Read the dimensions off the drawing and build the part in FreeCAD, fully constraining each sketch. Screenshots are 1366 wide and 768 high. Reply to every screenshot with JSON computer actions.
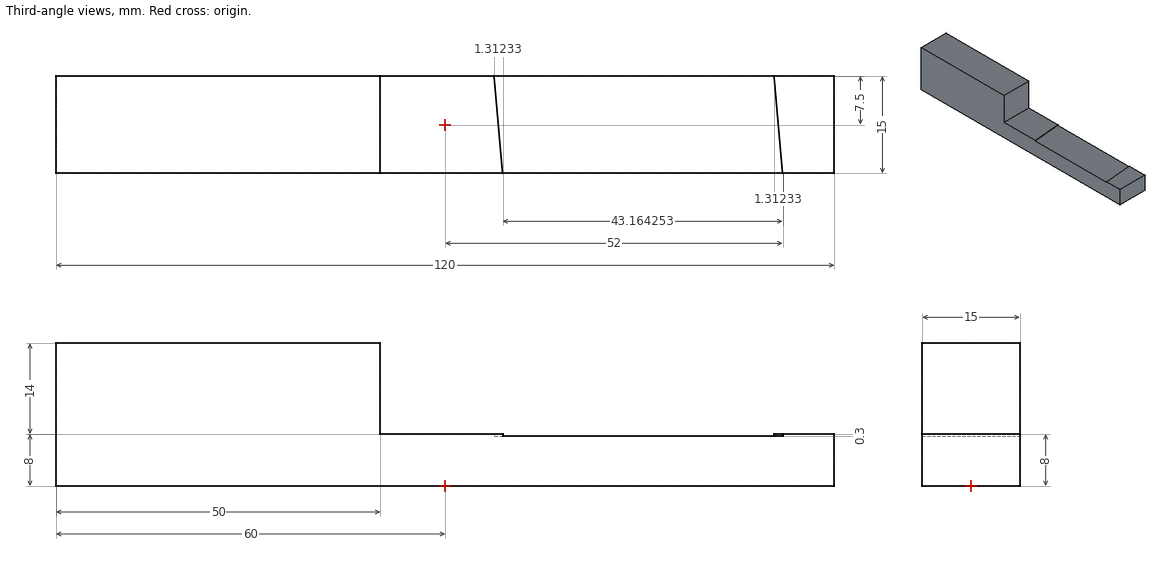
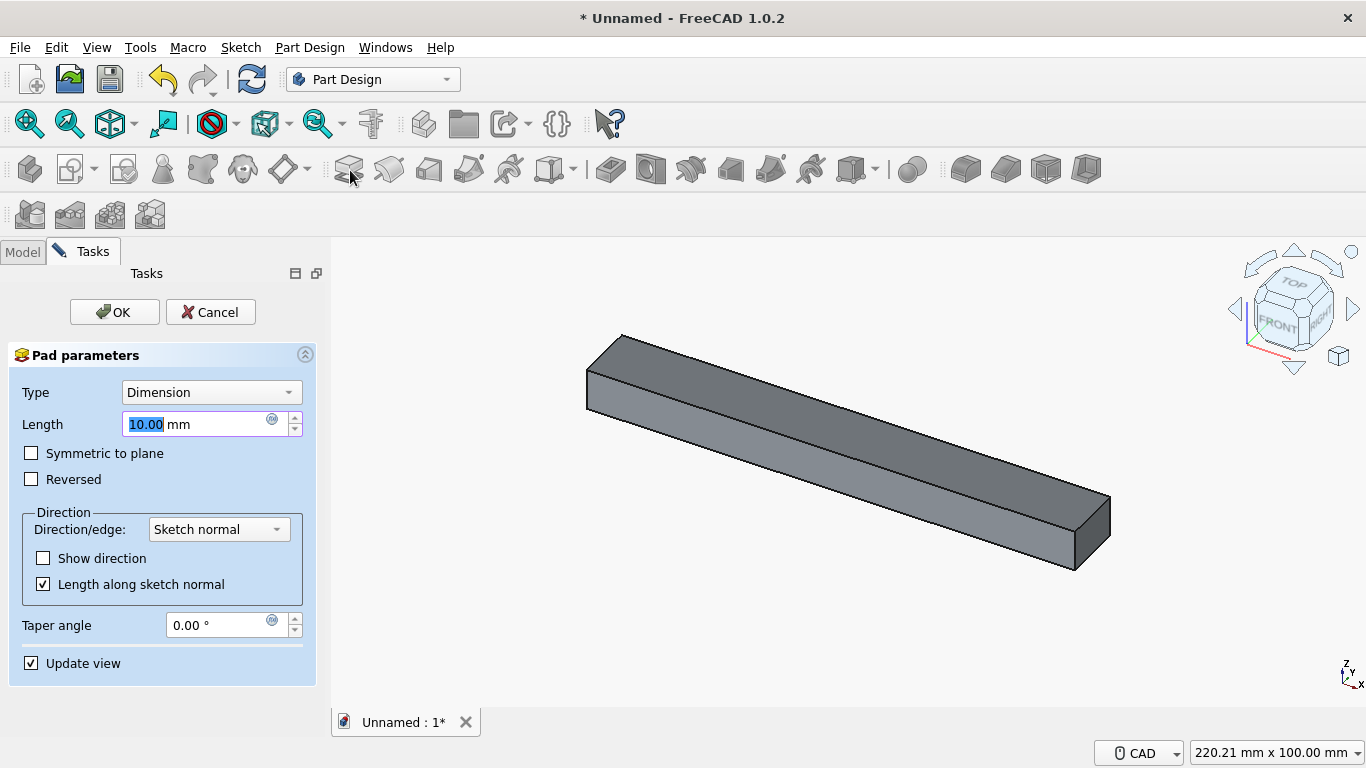
{"action": "type", "text": "8"}
{"action": "key", "text": "Tab"}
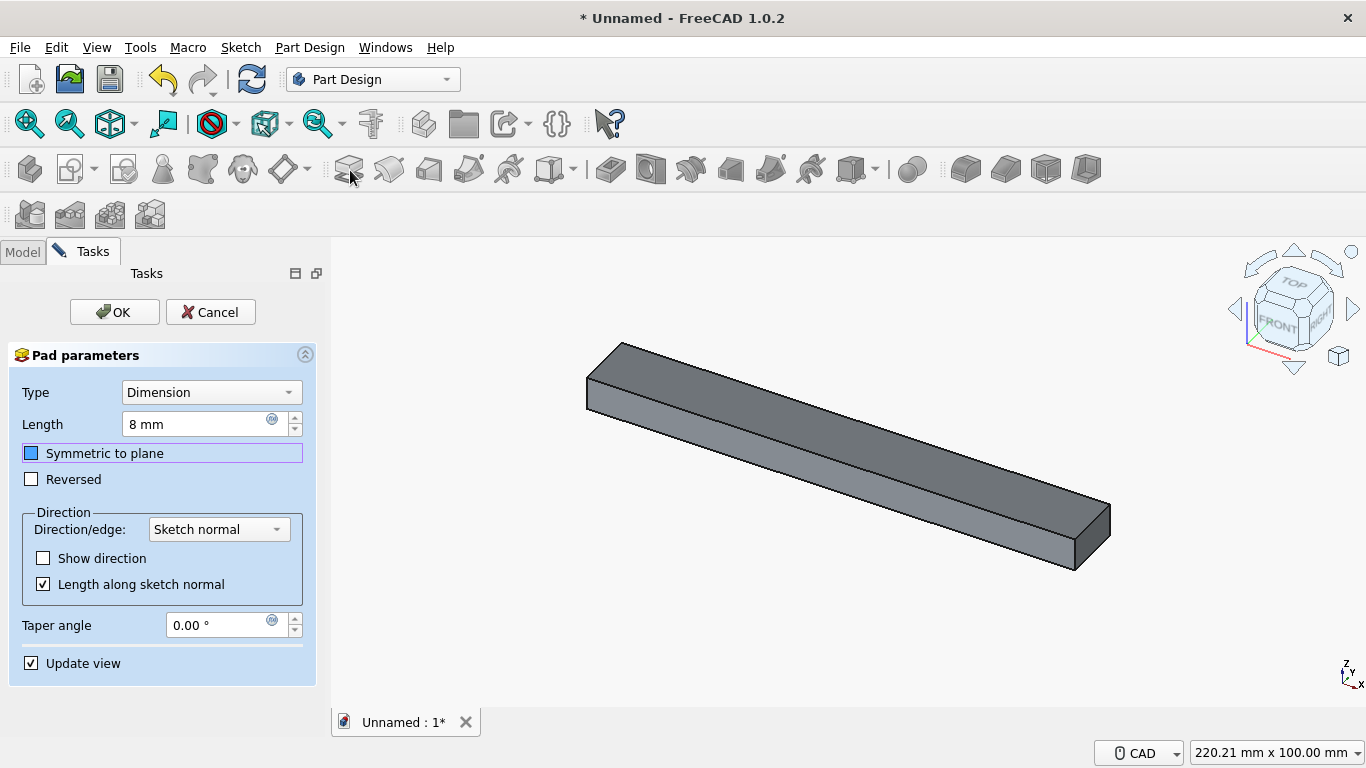
{"action": "left_click", "coordinate": [115, 312]}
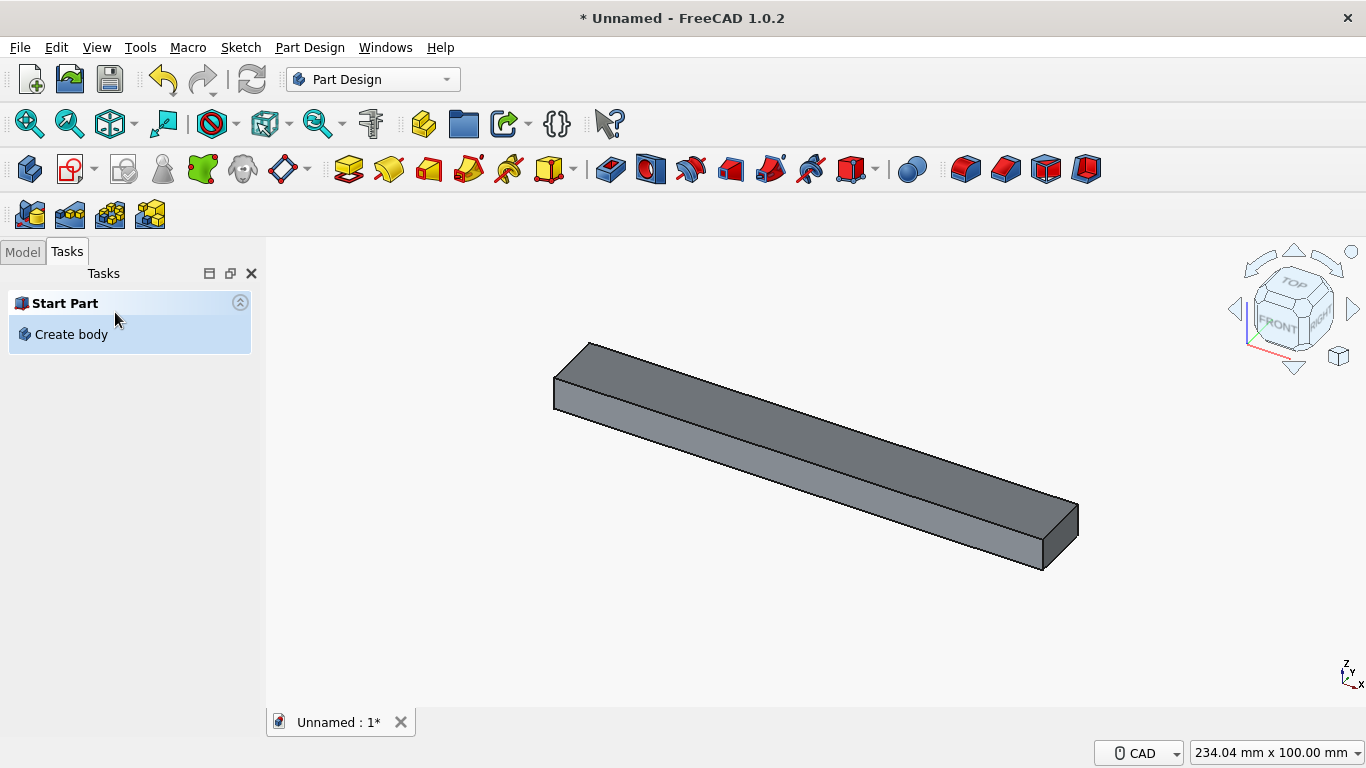
{"action": "left_click", "coordinate": [1025, 510]}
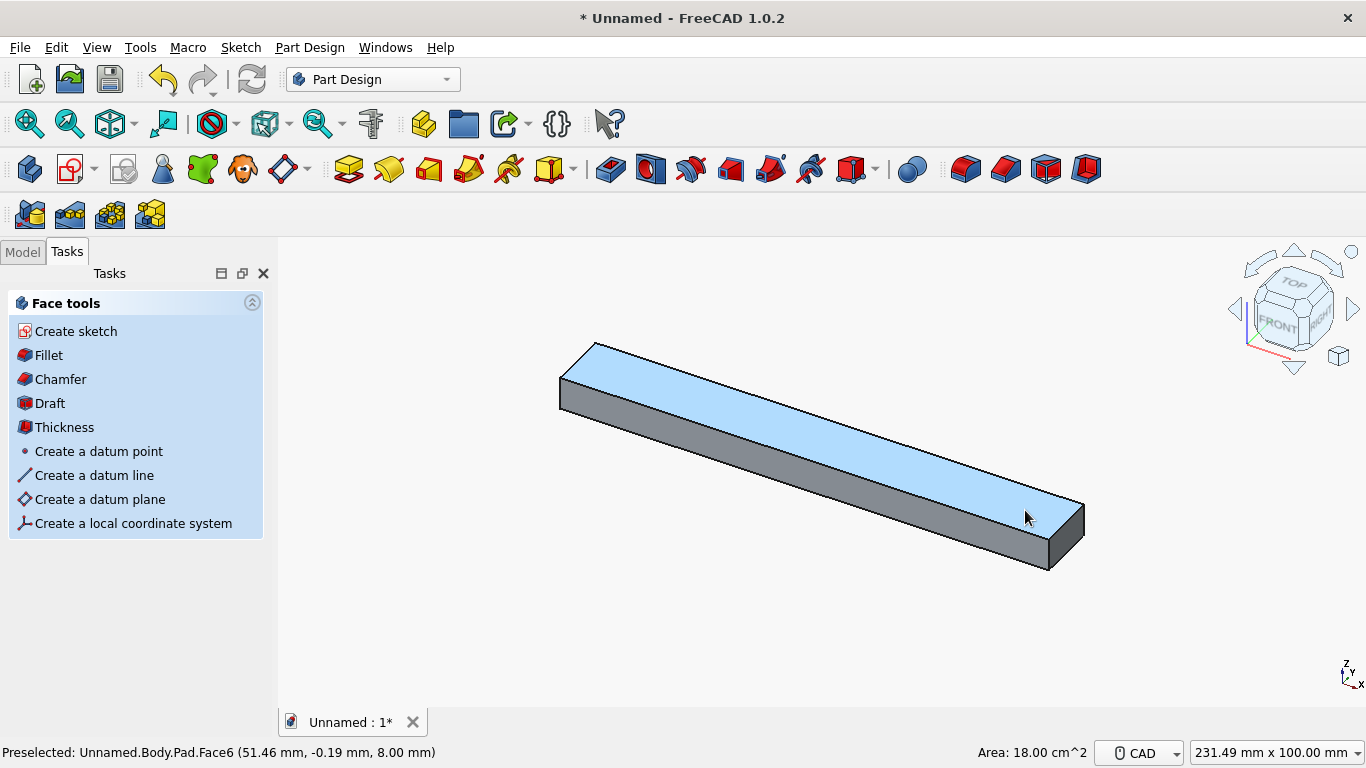
{"action": "left_click", "coordinate": [70, 170]}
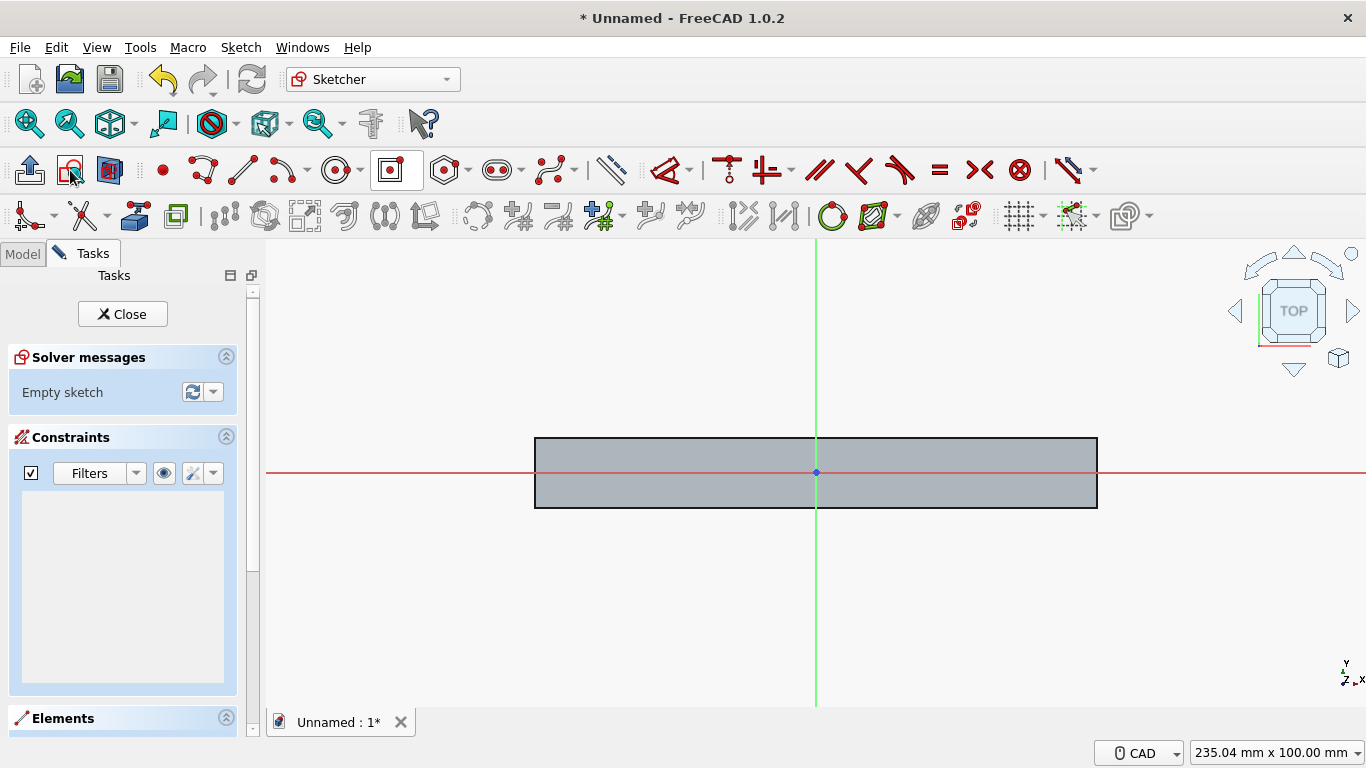
{"action": "scroll", "coordinate": [1048, 473], "scroll_direction": "up", "scroll_amount": 5}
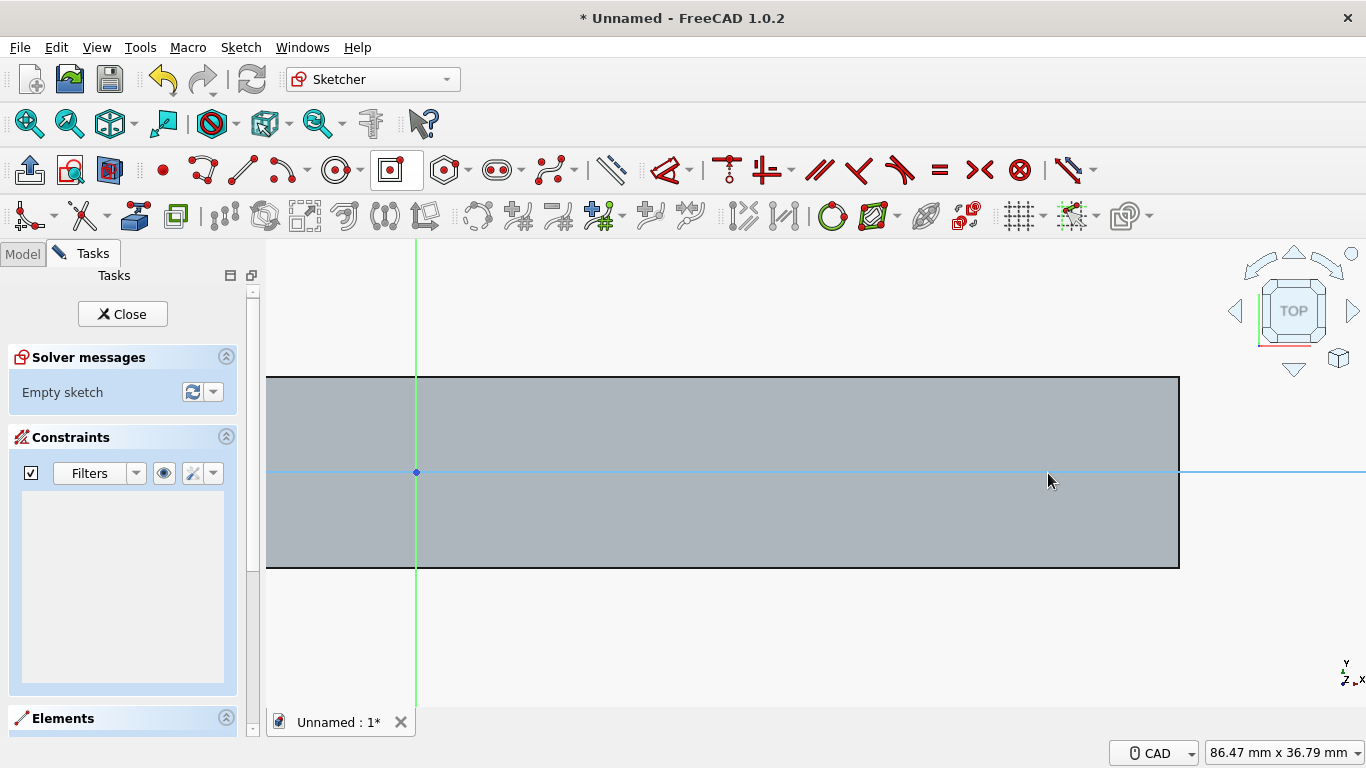
{"action": "left_click", "coordinate": [204, 170]}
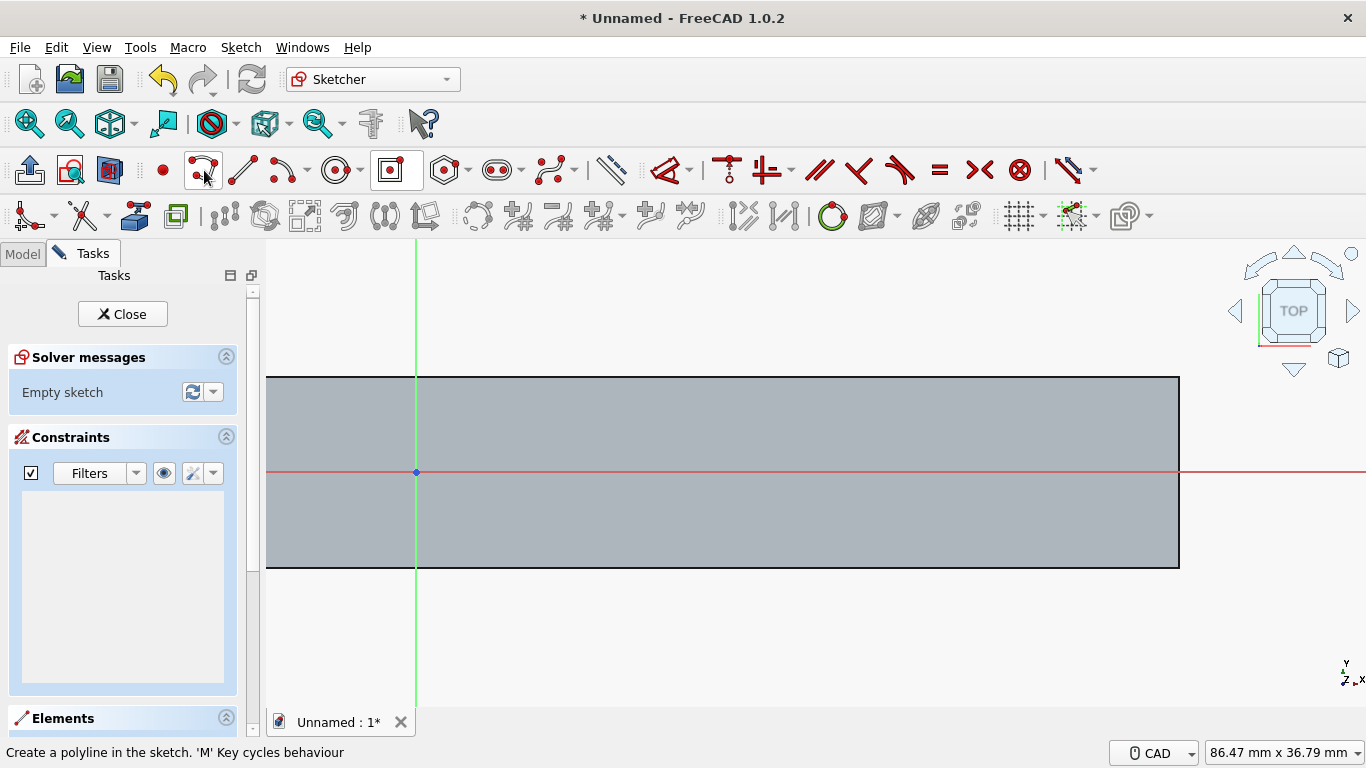
{"action": "left_click", "coordinate": [512, 377]}
{"action": "left_click", "coordinate": [529, 568]}
{"action": "left_click", "coordinate": [1078, 568]}
{"action": "left_click", "coordinate": [1061, 377]}
{"action": "left_click", "coordinate": [512, 378]}
{"action": "key", "text": "Escape"}
{"action": "key", "text": "Escape"}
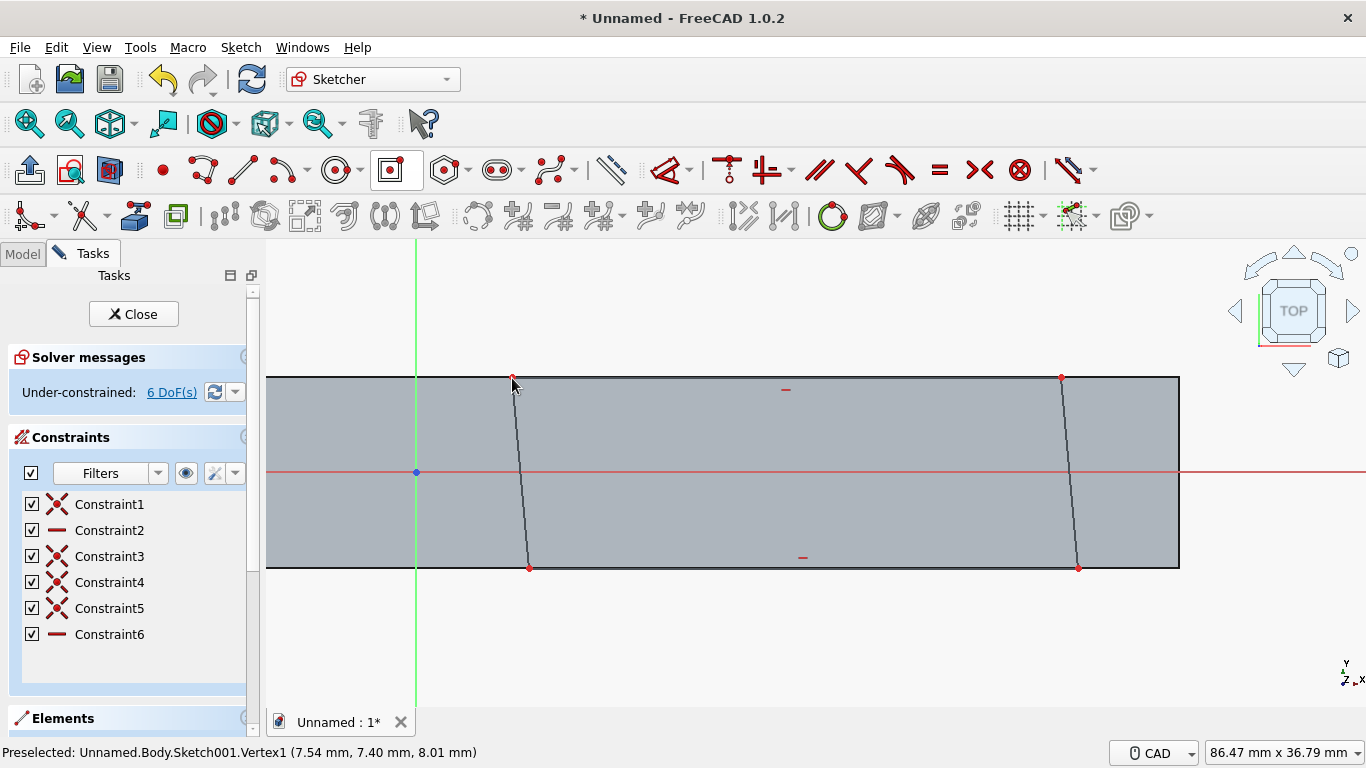
{"action": "left_click", "coordinate": [666, 170]}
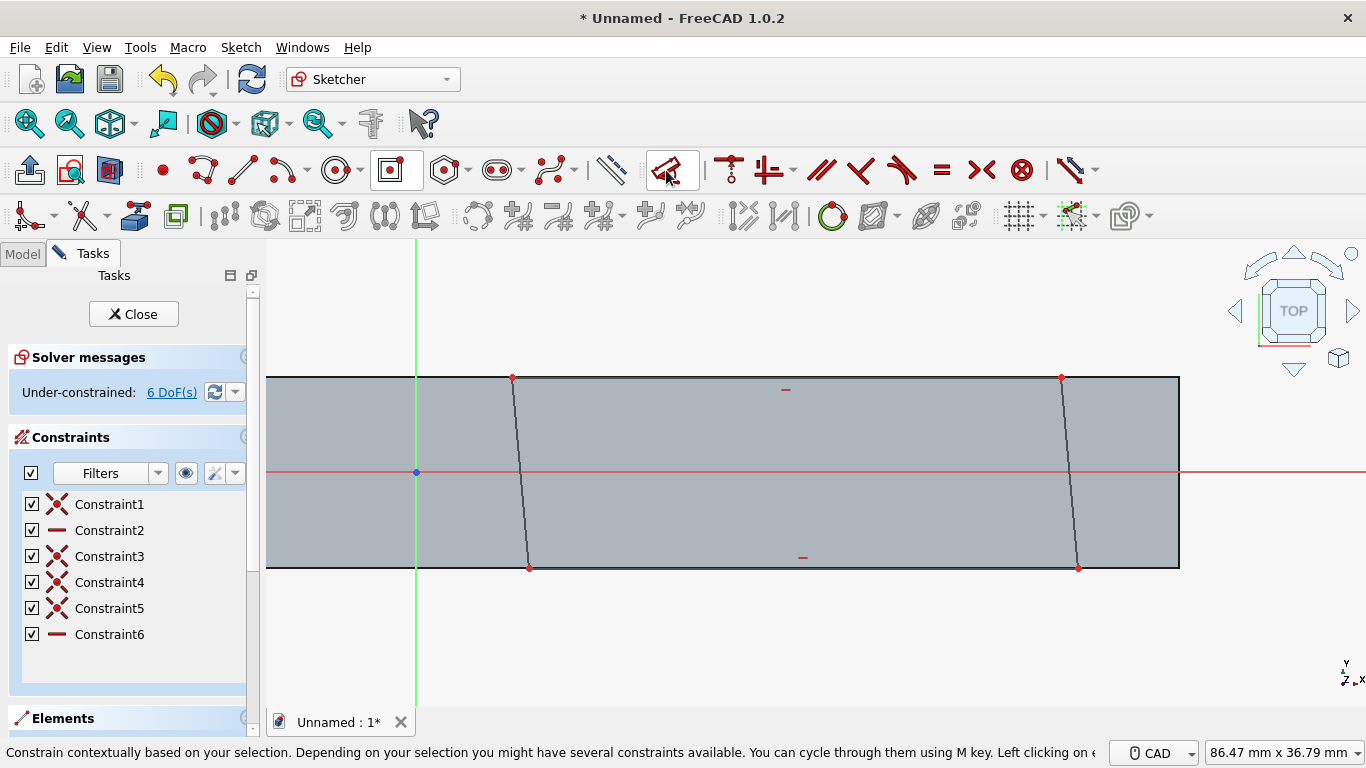
{"action": "left_click", "coordinate": [1078, 569]}
{"action": "left_click", "coordinate": [747, 603]}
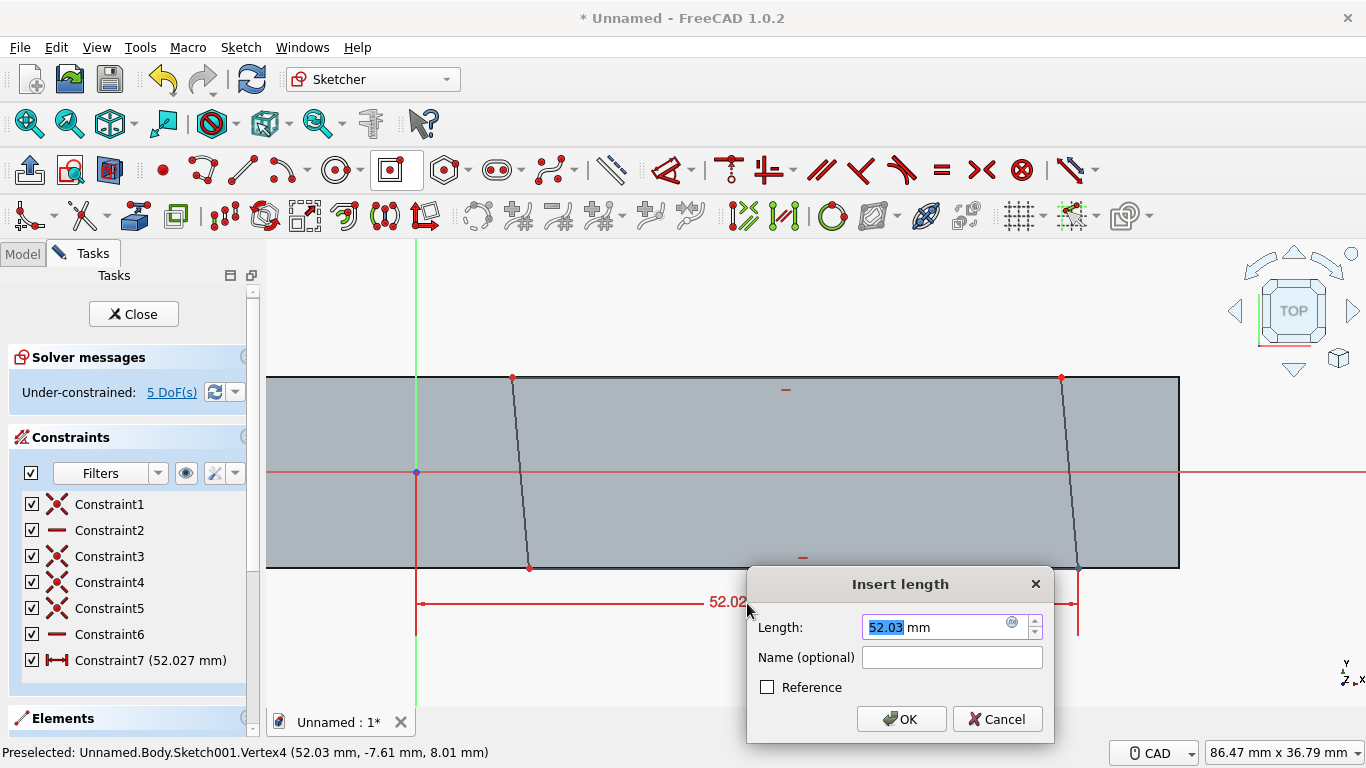
{"action": "type", "text": "52"}
{"action": "key", "text": "Return"}